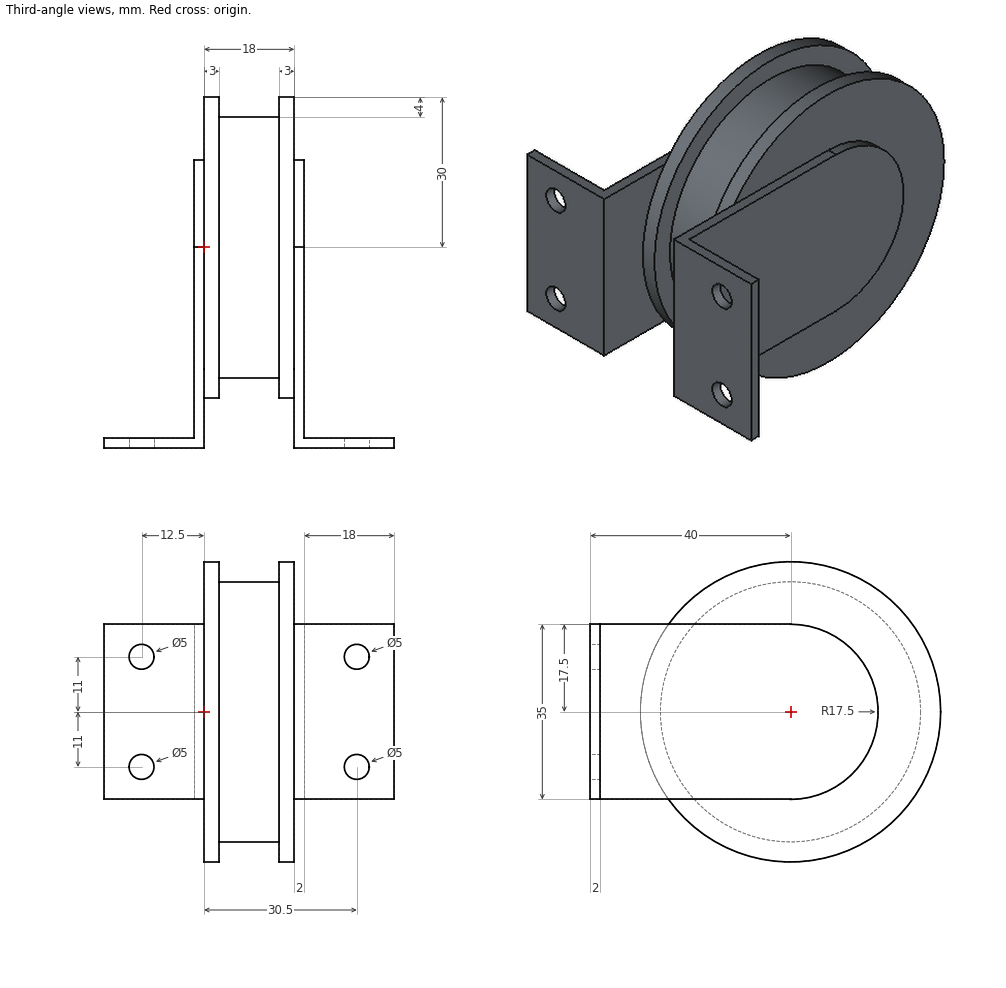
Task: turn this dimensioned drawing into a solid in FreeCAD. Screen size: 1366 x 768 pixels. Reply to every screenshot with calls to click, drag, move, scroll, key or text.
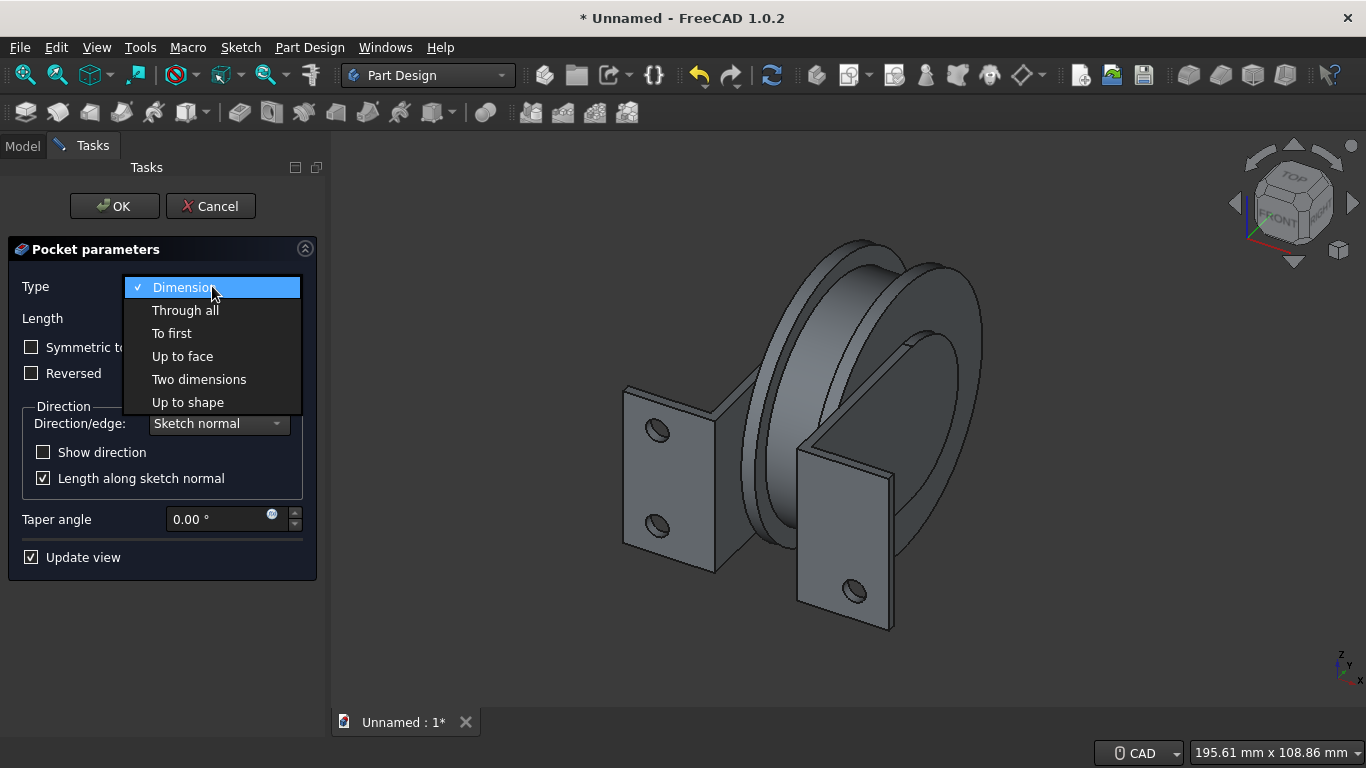
click(212, 334)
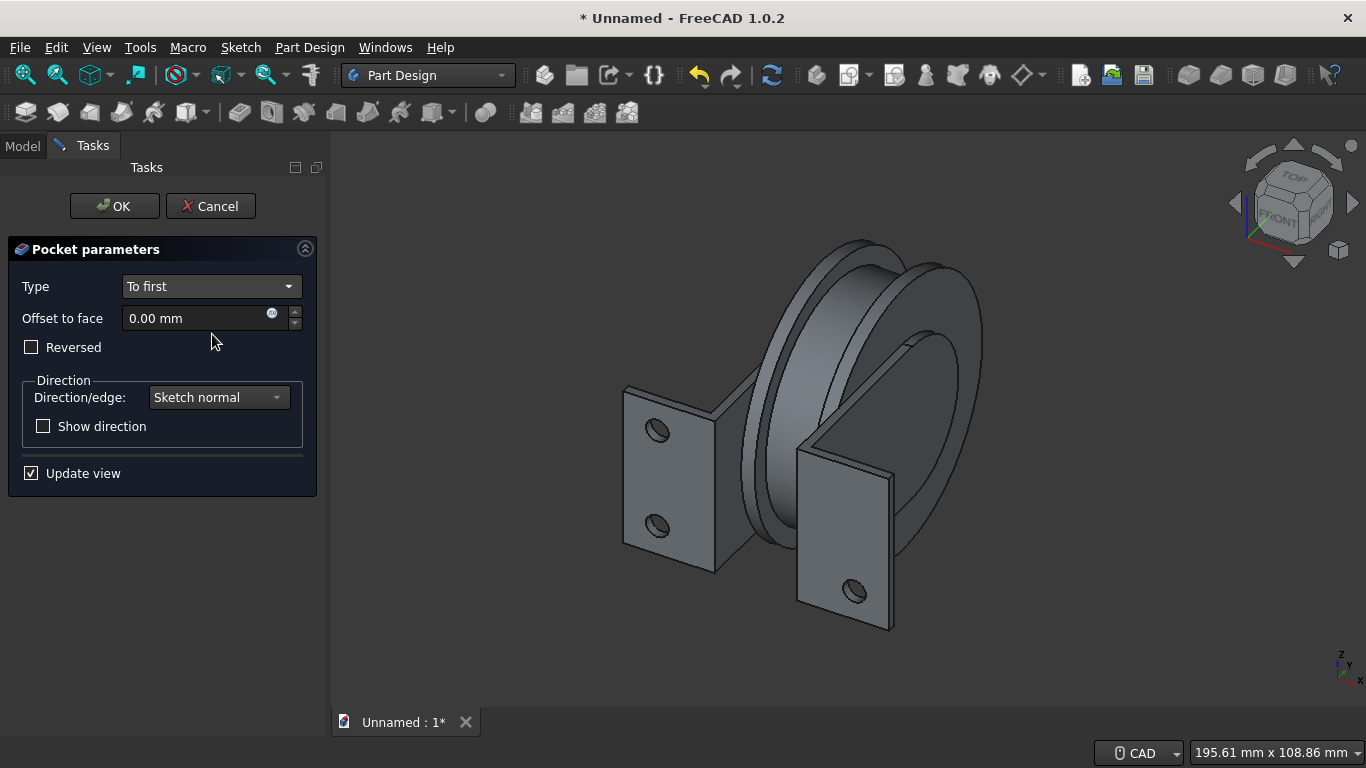
click(115, 206)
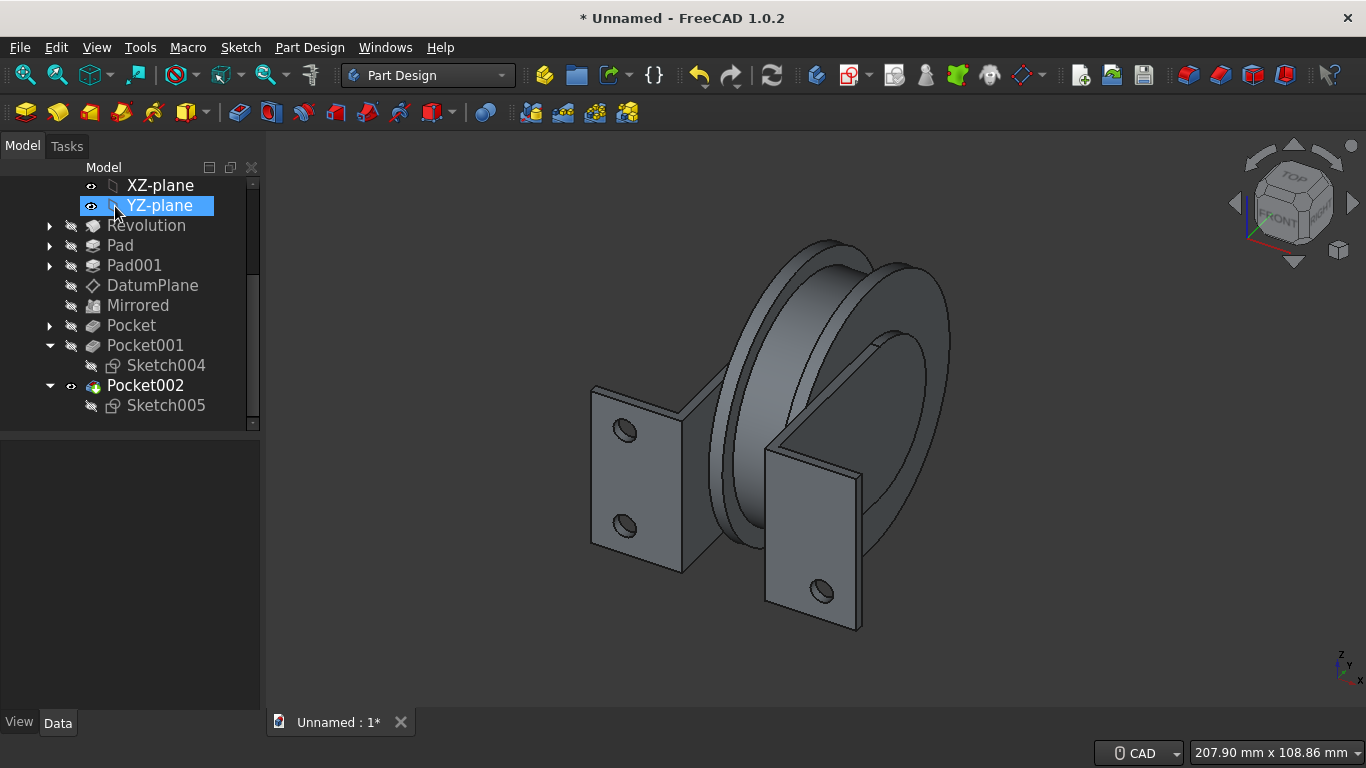
click(810, 517)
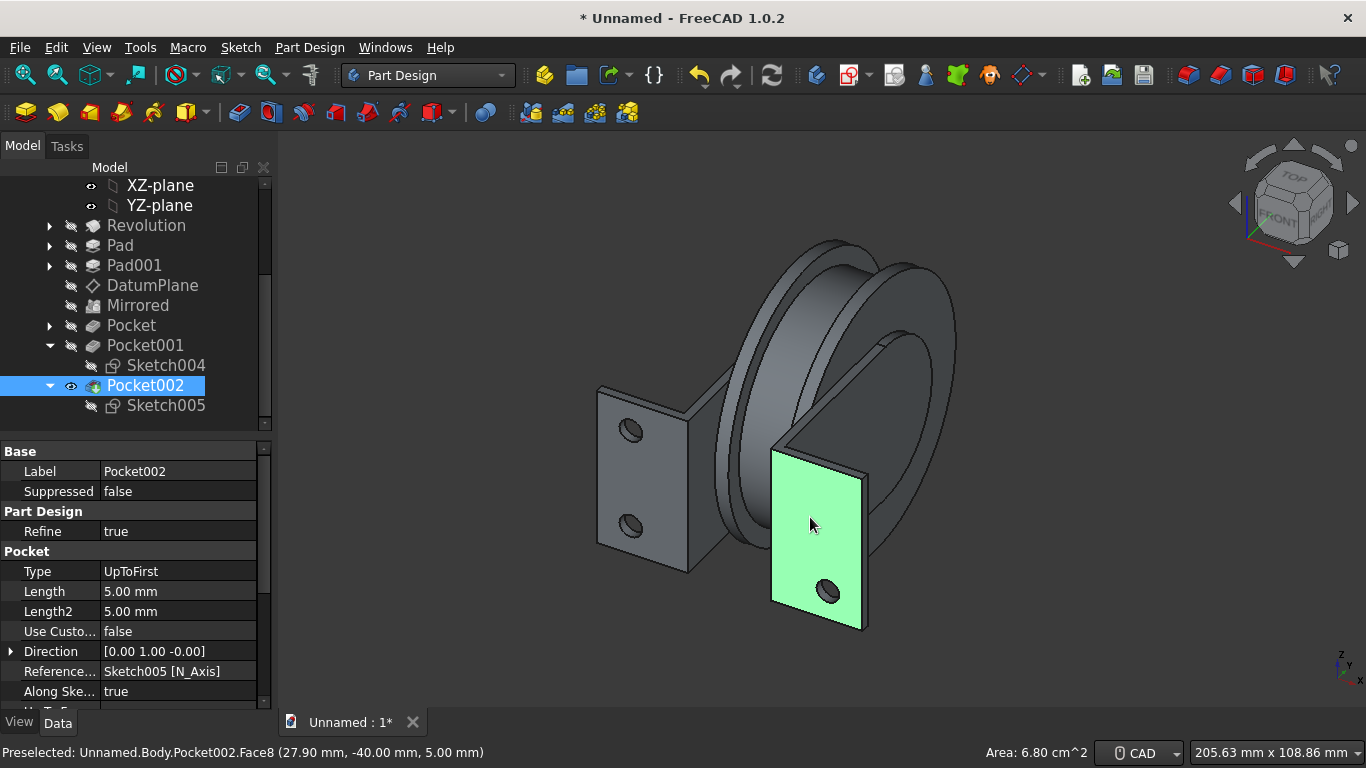
click(850, 76)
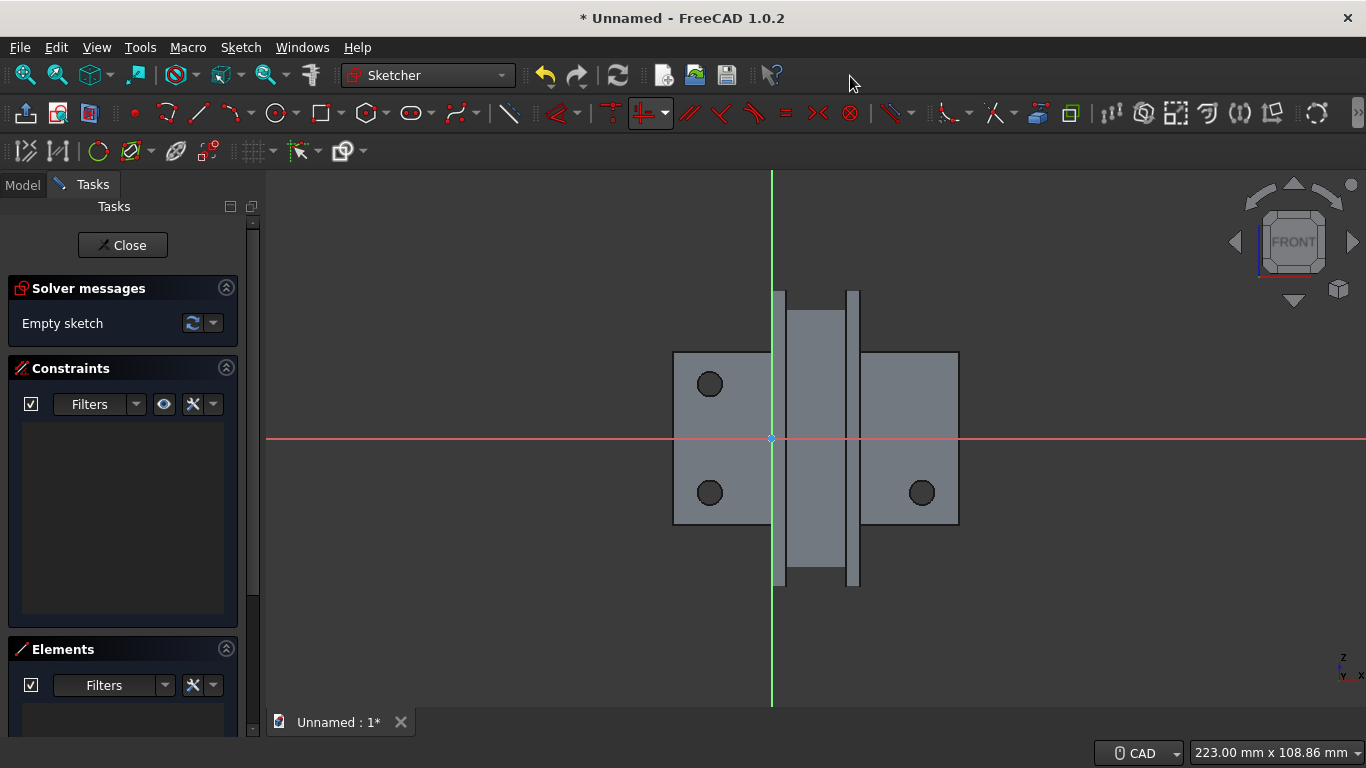
scroll(936, 380, up, 13)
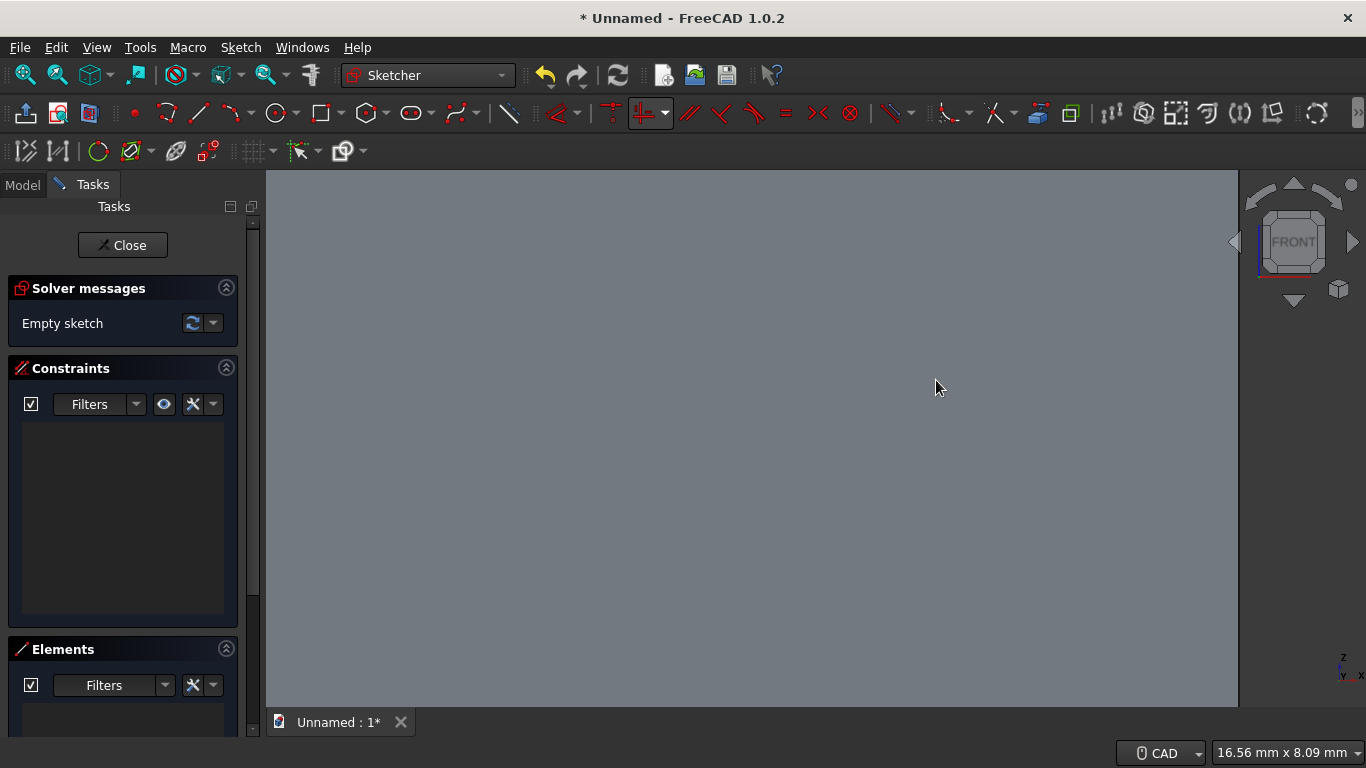
key(g)
key(c)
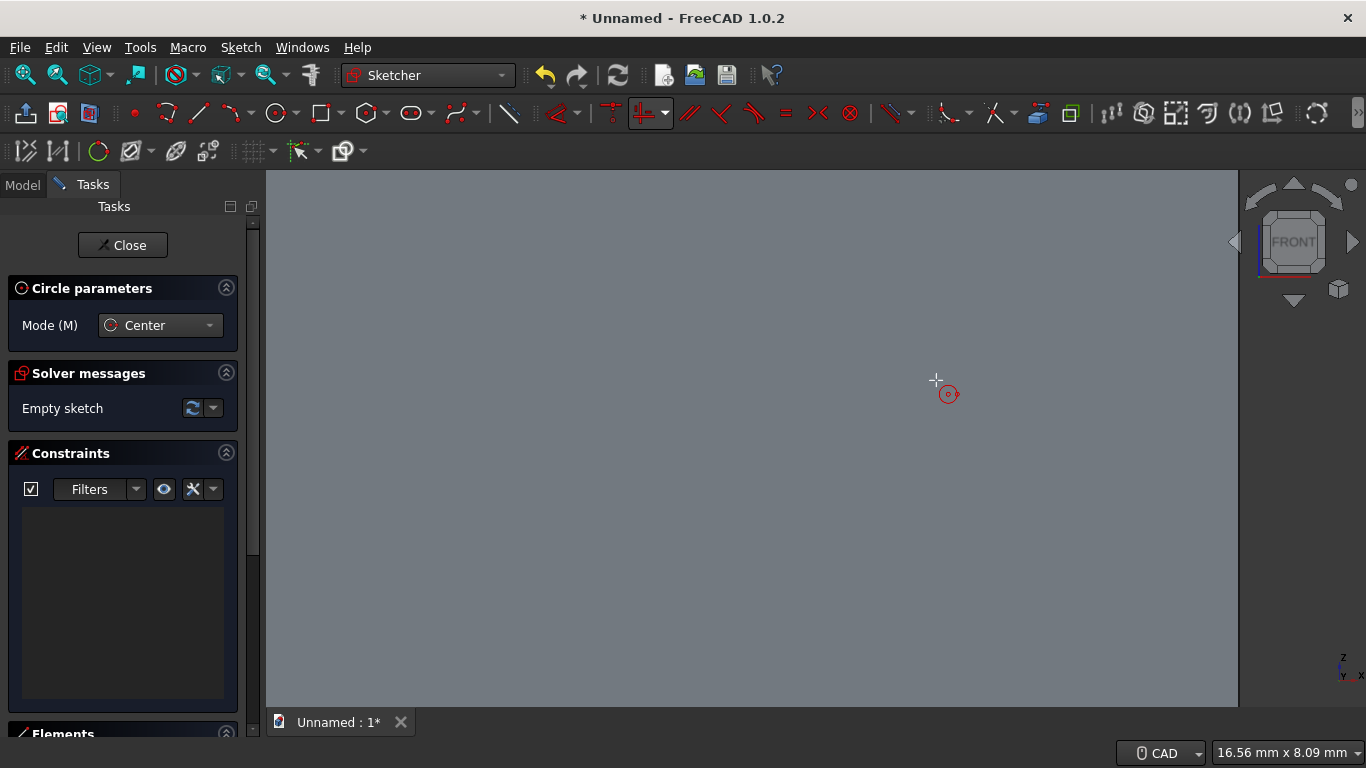
click(741, 432)
click(858, 315)
key(Escape)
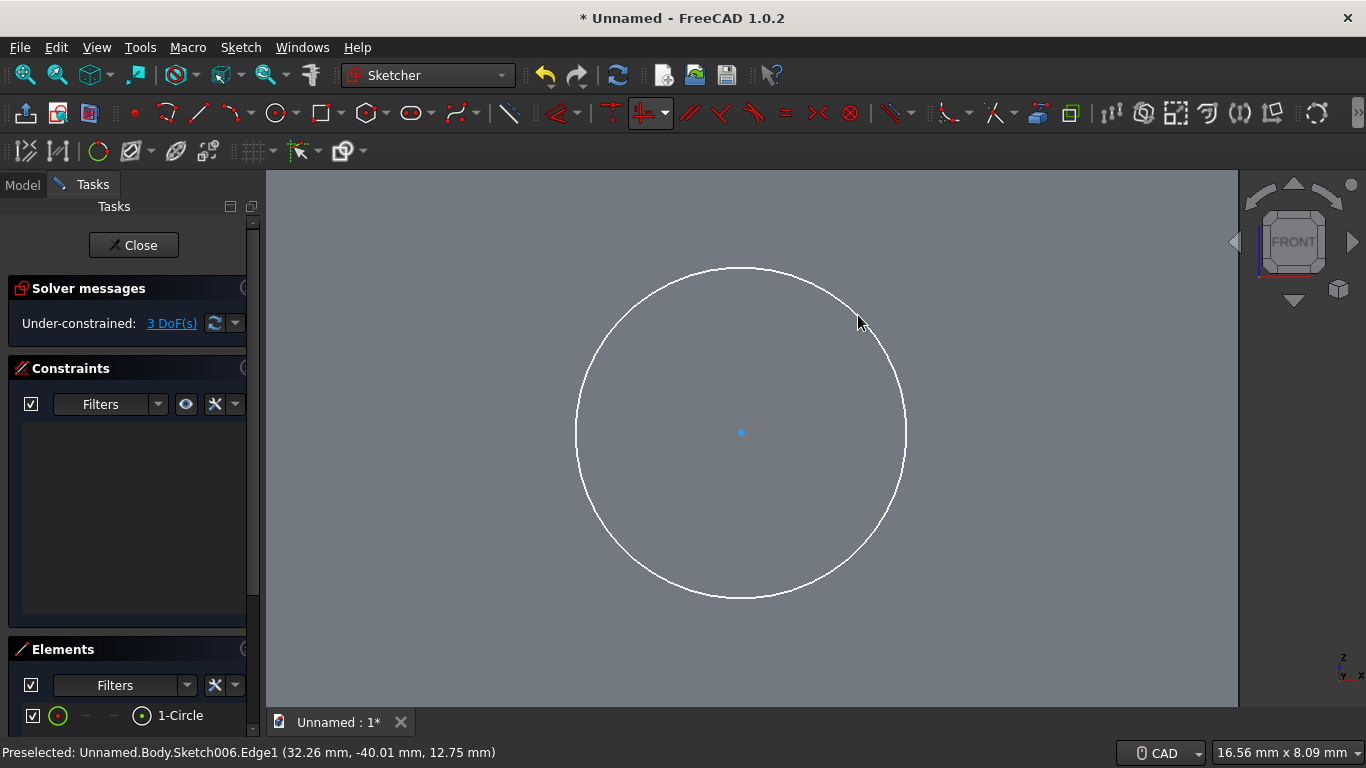
click(556, 114)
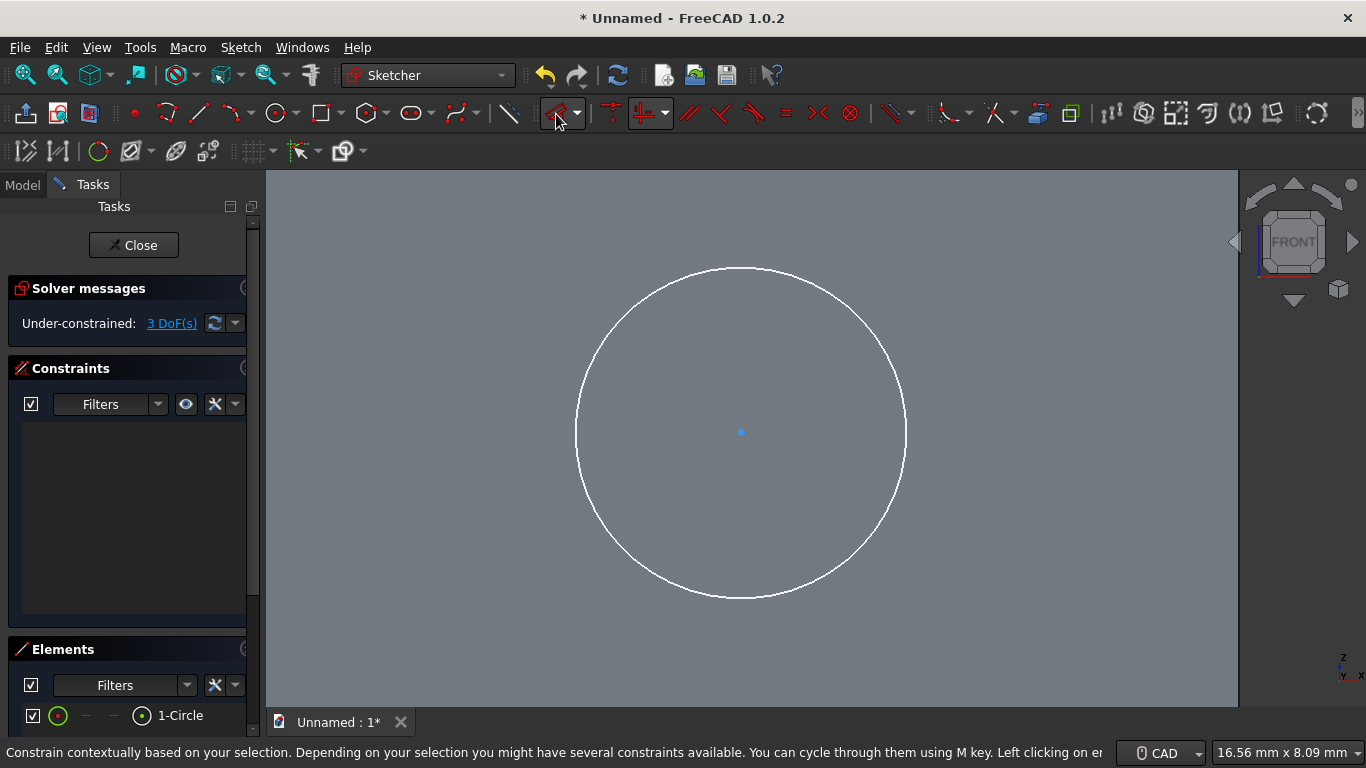
click(858, 316)
click(881, 293)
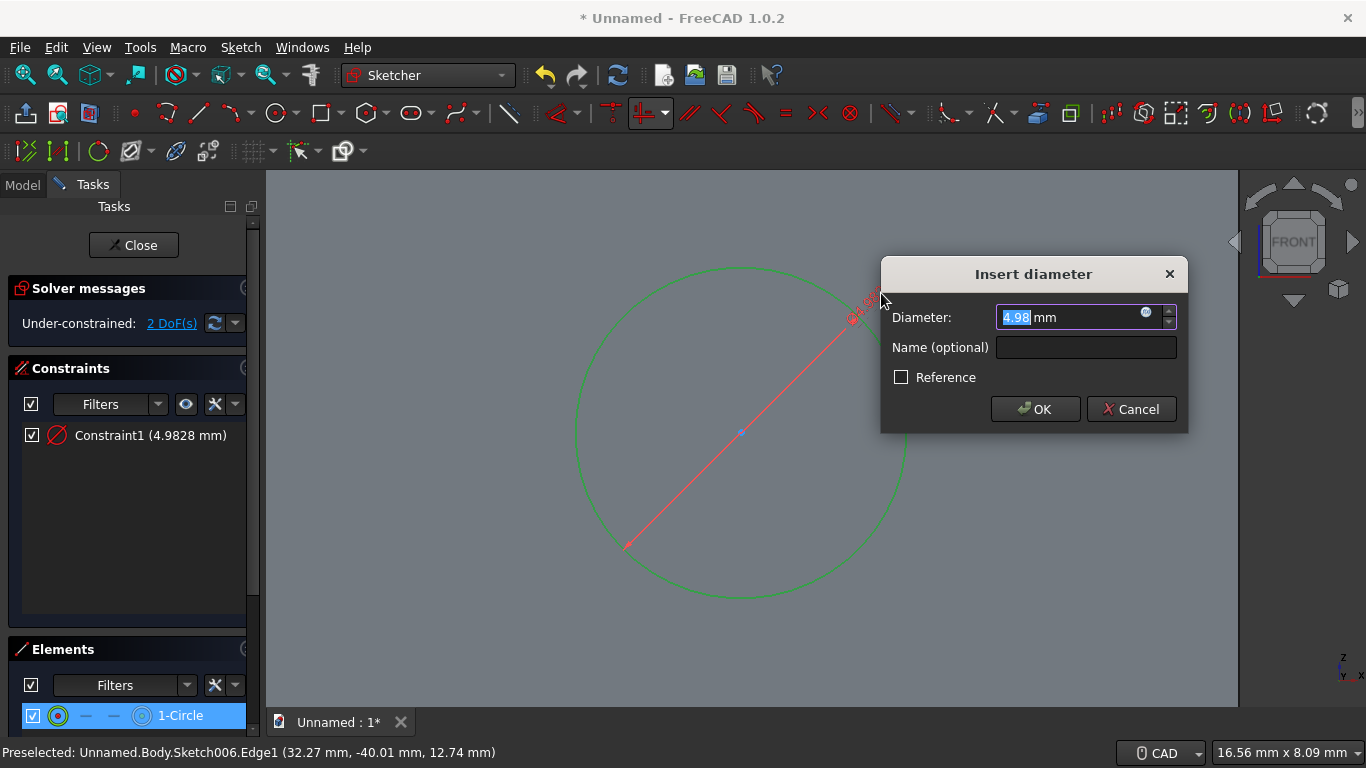
text(5)
key(Return)